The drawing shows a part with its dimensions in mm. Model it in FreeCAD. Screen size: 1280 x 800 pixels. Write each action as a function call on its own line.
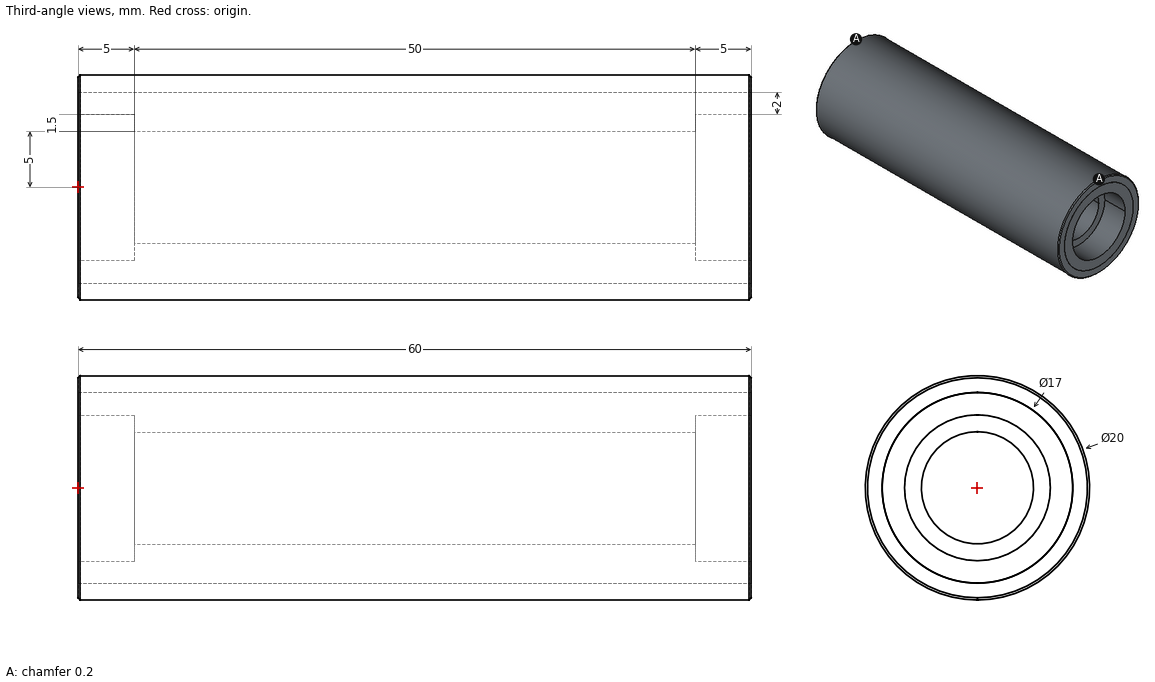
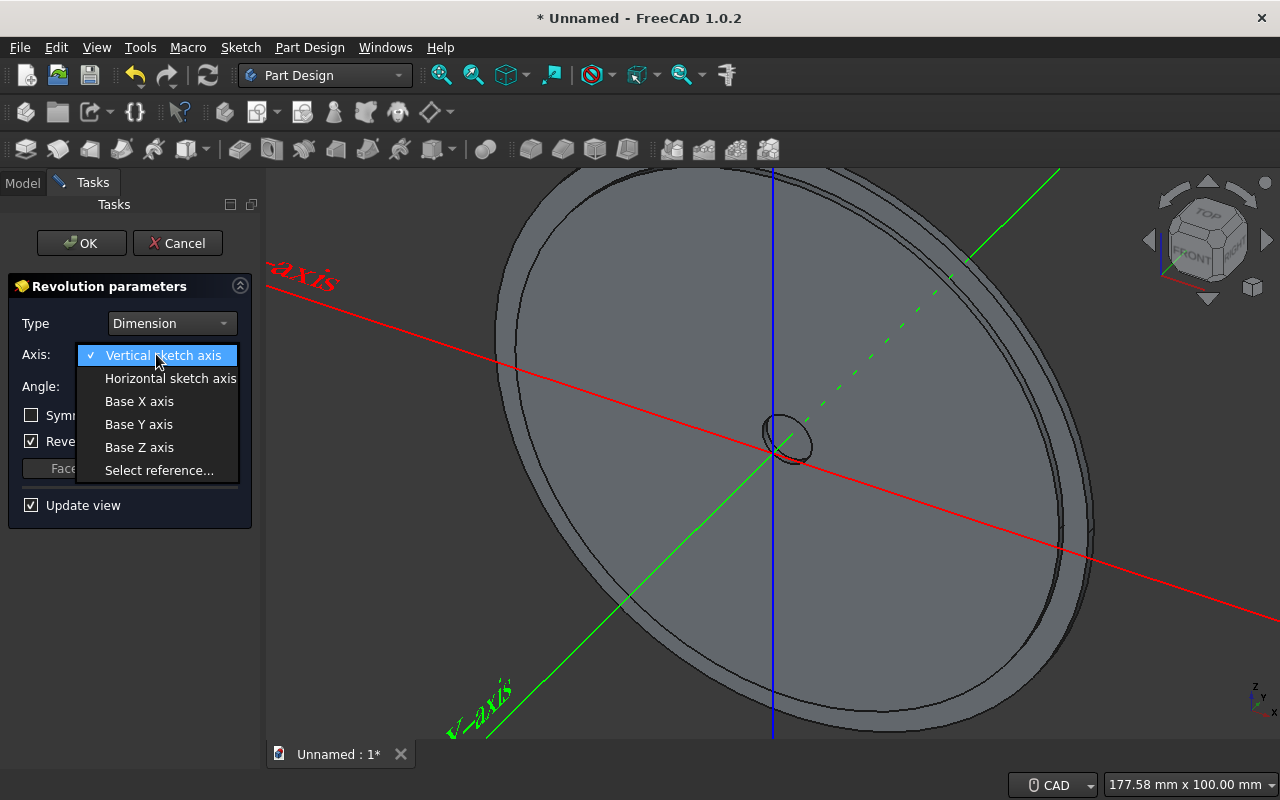
click(156, 378)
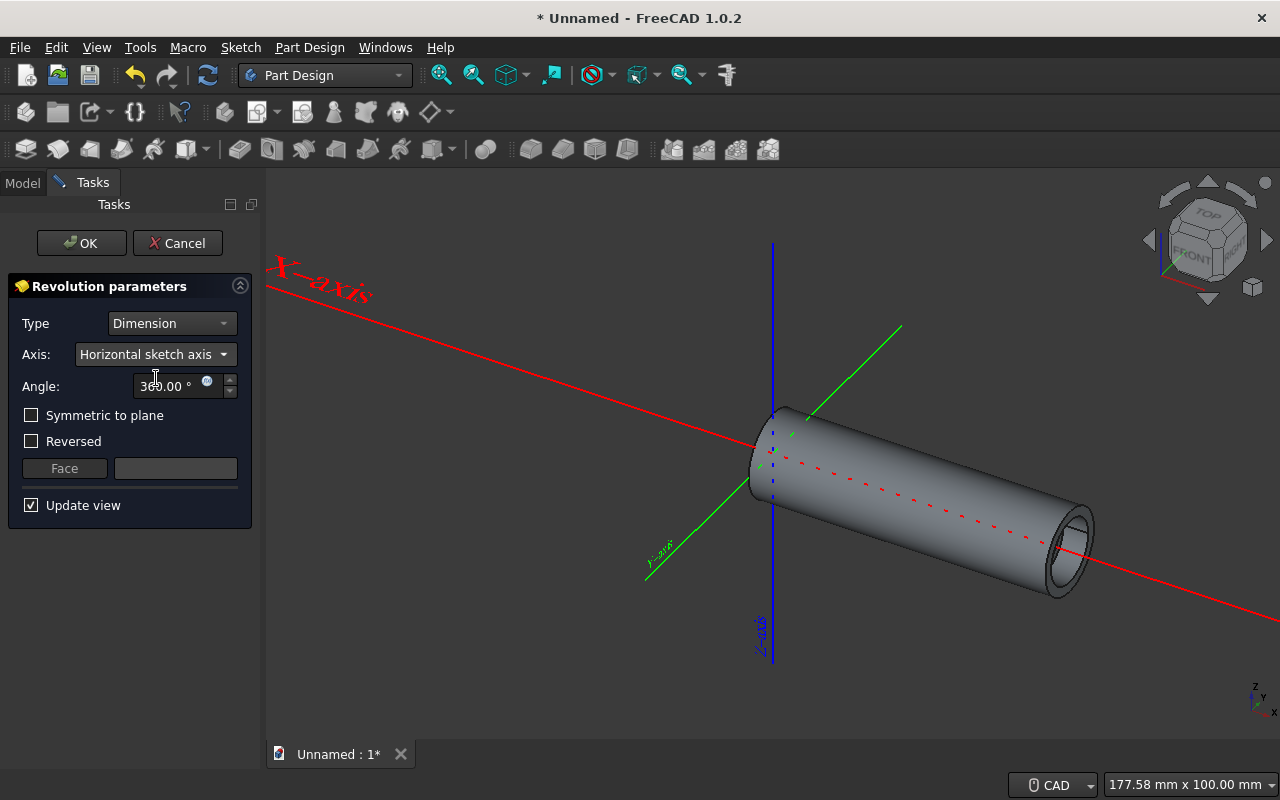
click(82, 243)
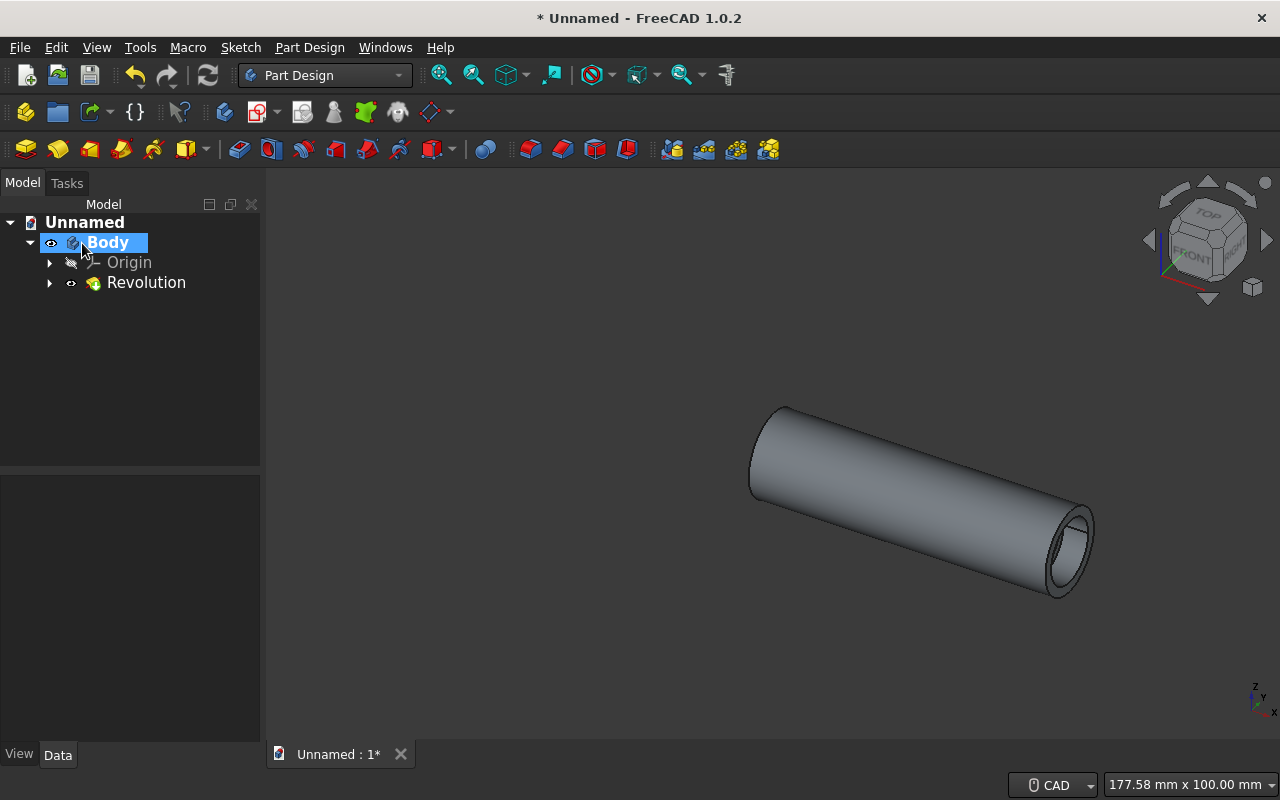
click(442, 76)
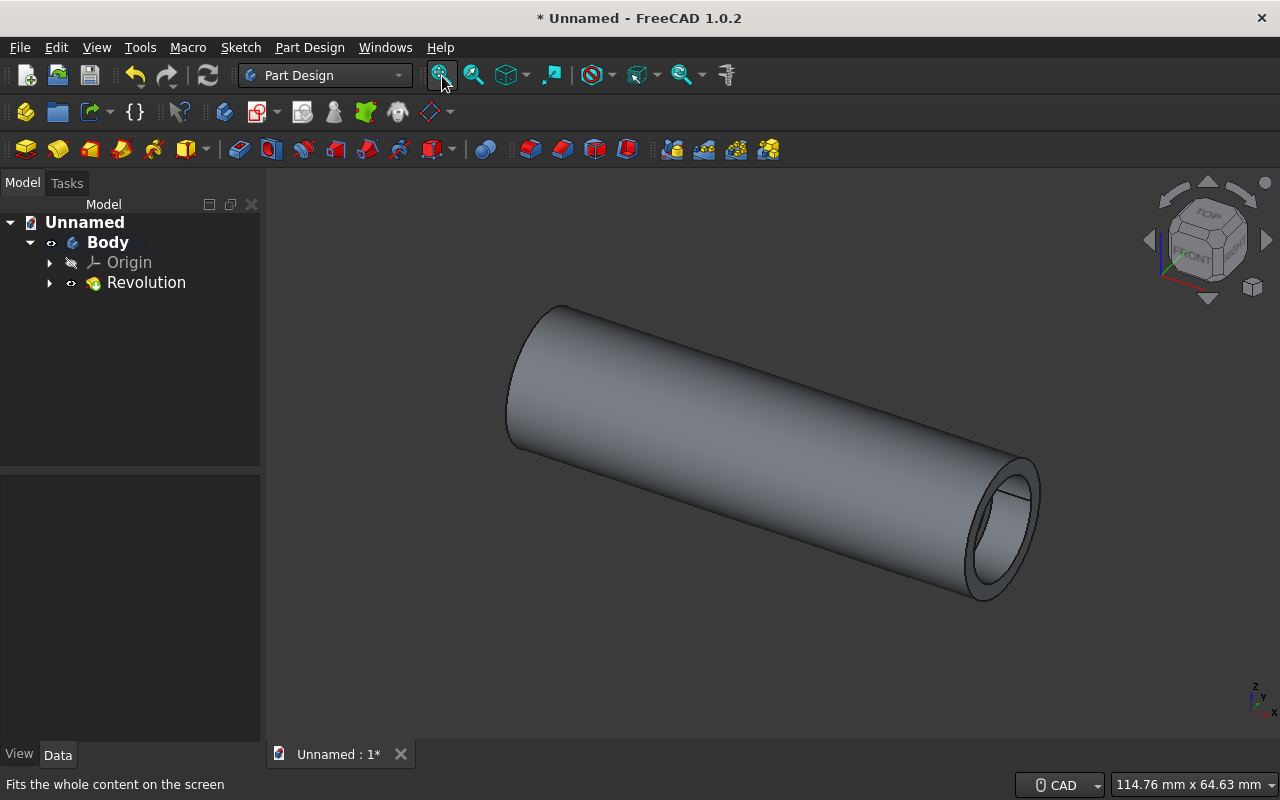
click(226, 112)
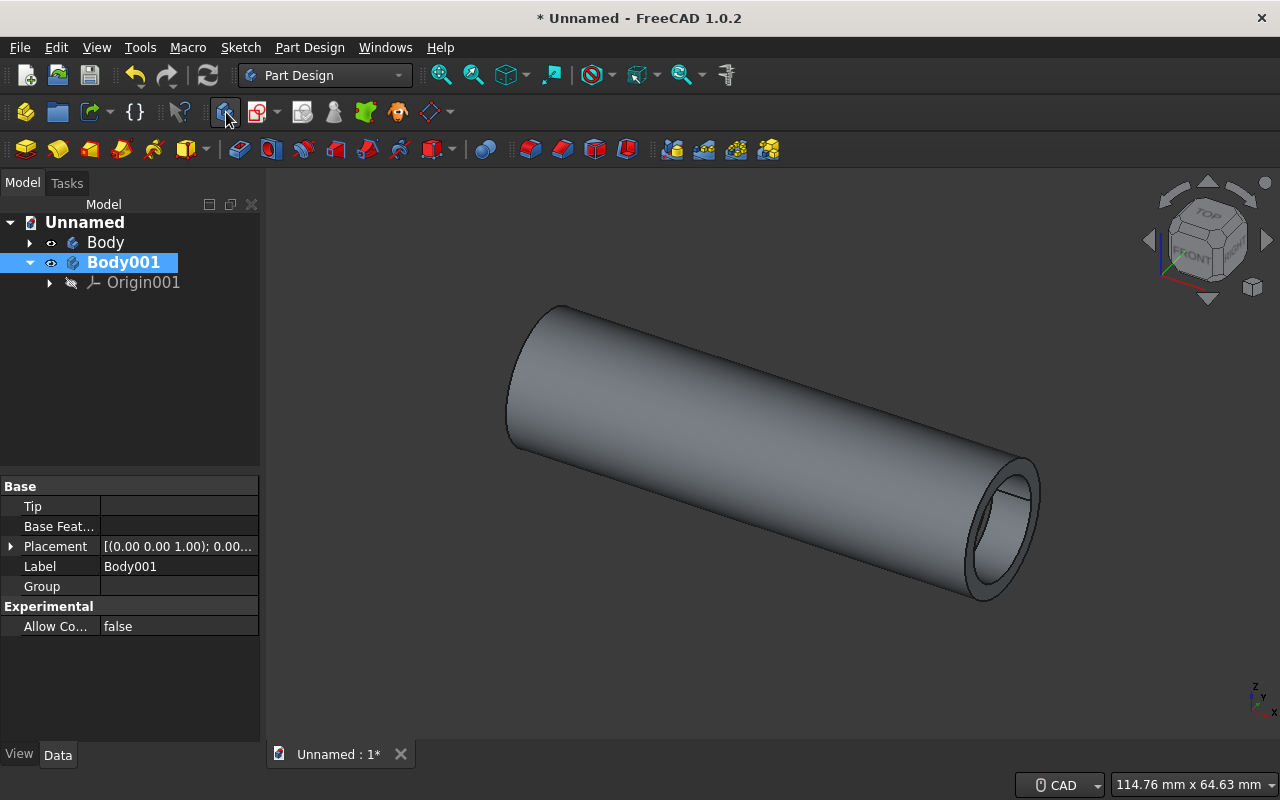
click(50, 283)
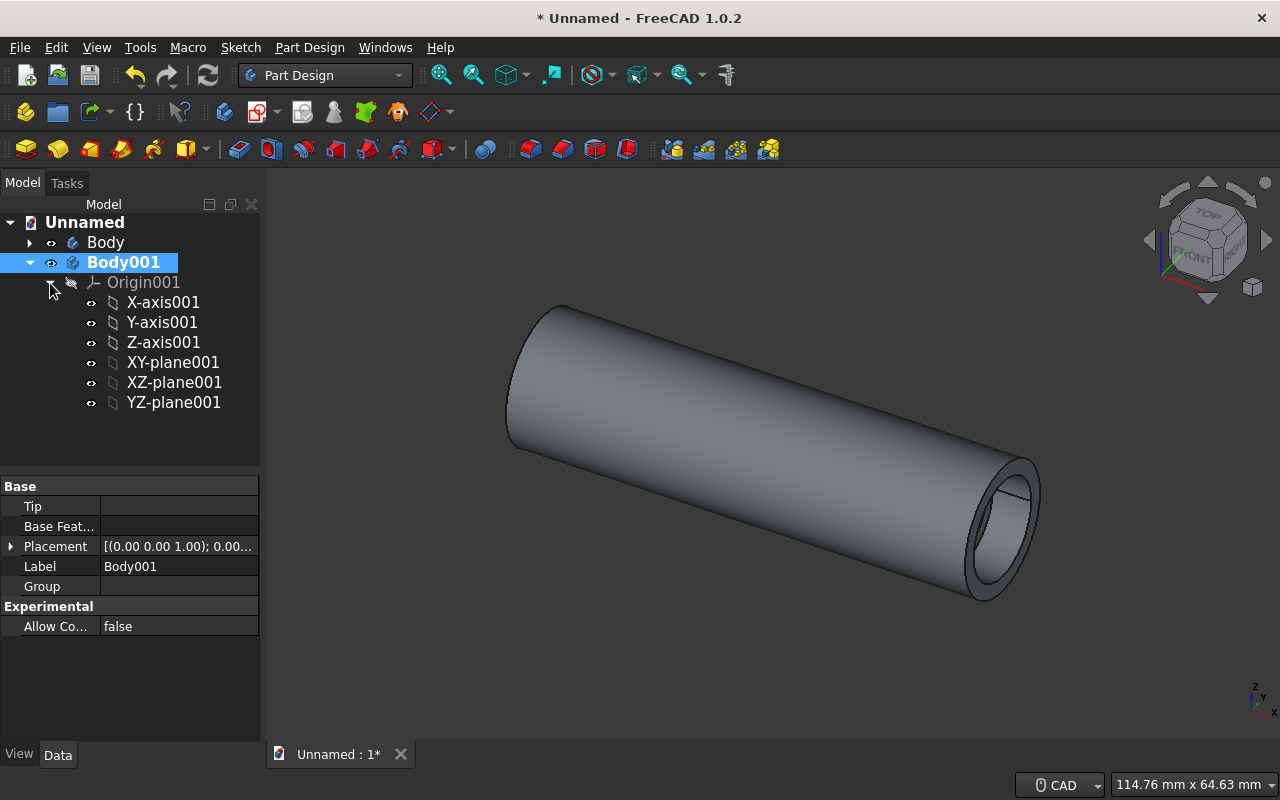
click(136, 403)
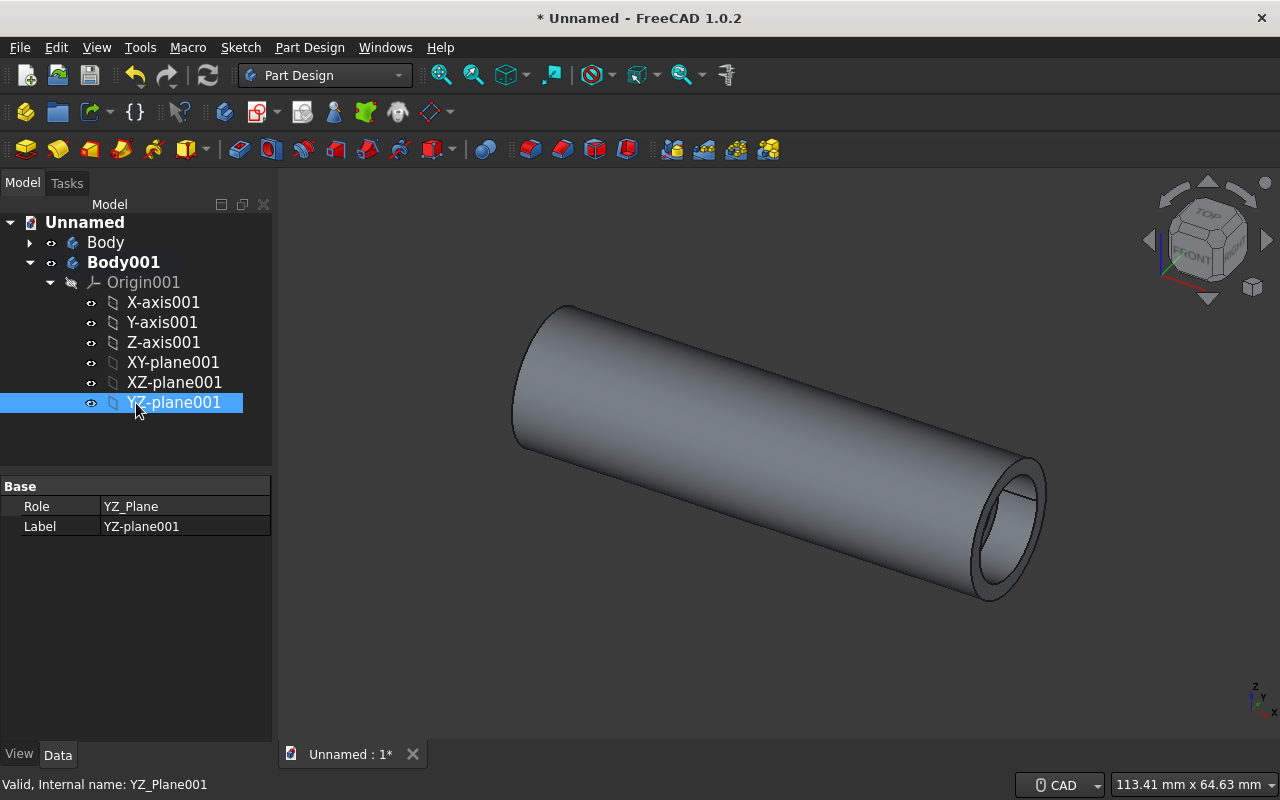
click(430, 112)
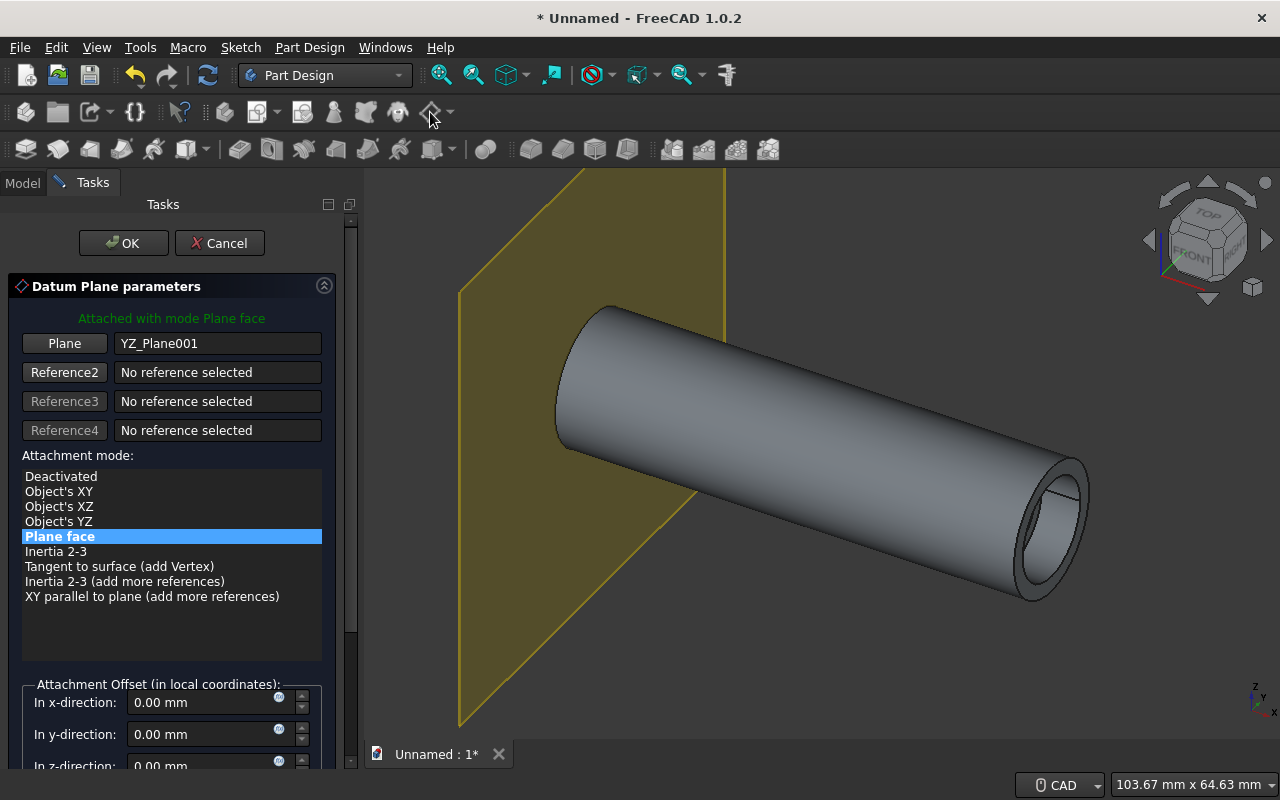
scroll(351, 491, down, 2)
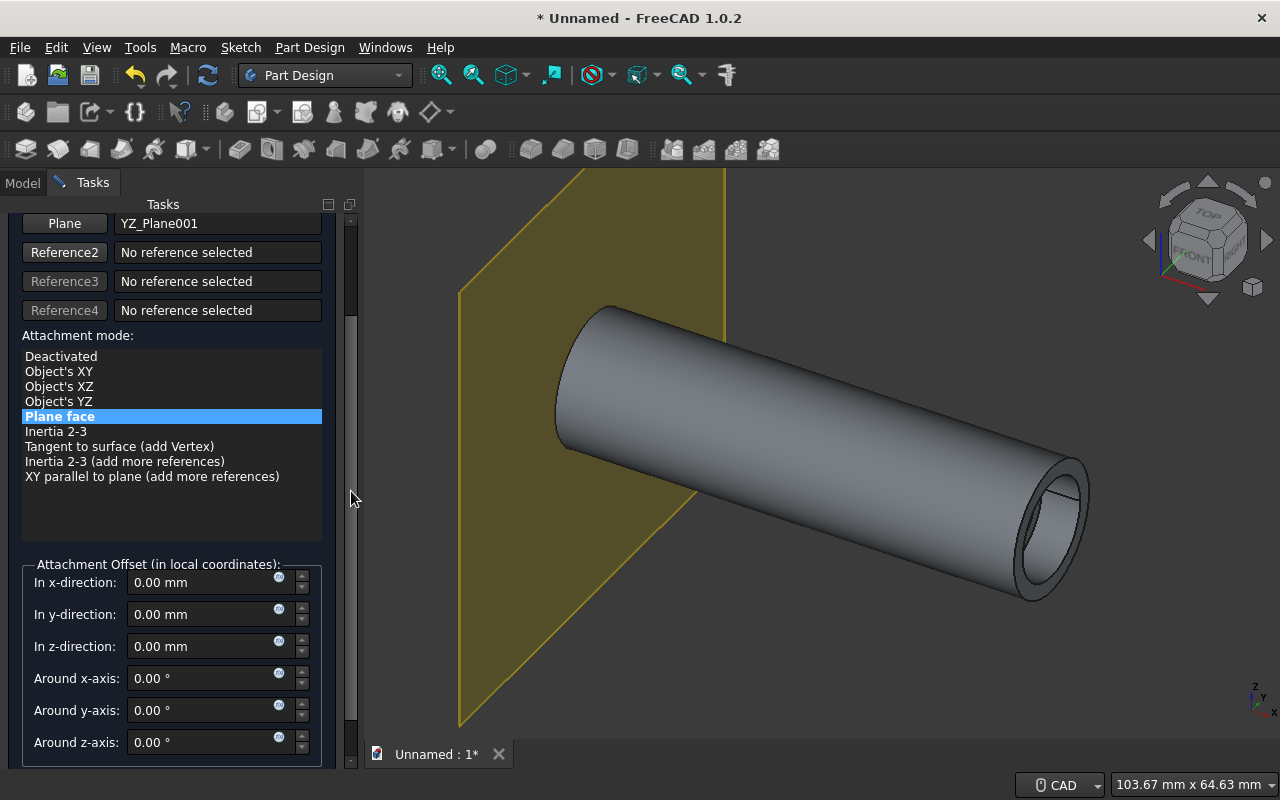
triple_click(210, 646)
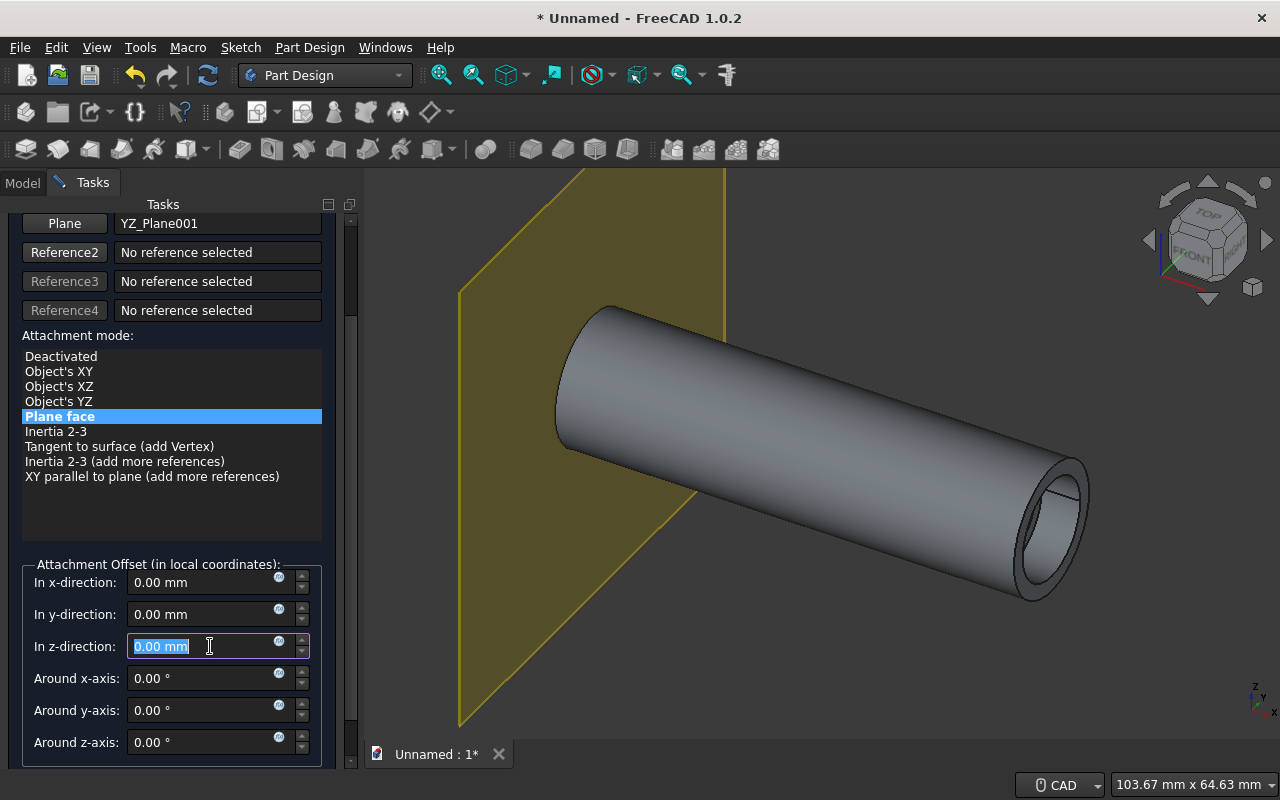
text(60)
key(Tab)